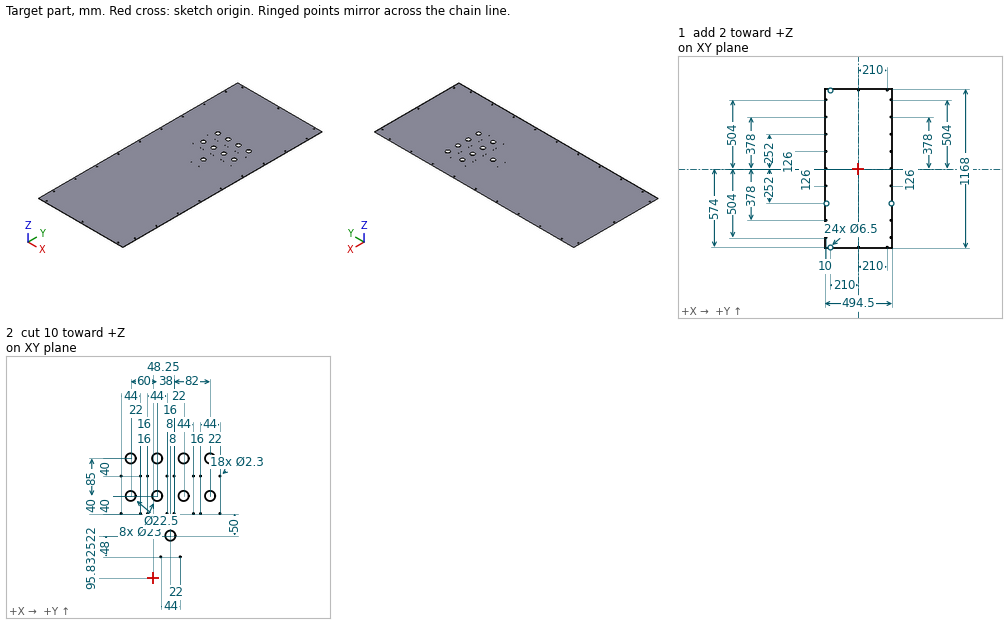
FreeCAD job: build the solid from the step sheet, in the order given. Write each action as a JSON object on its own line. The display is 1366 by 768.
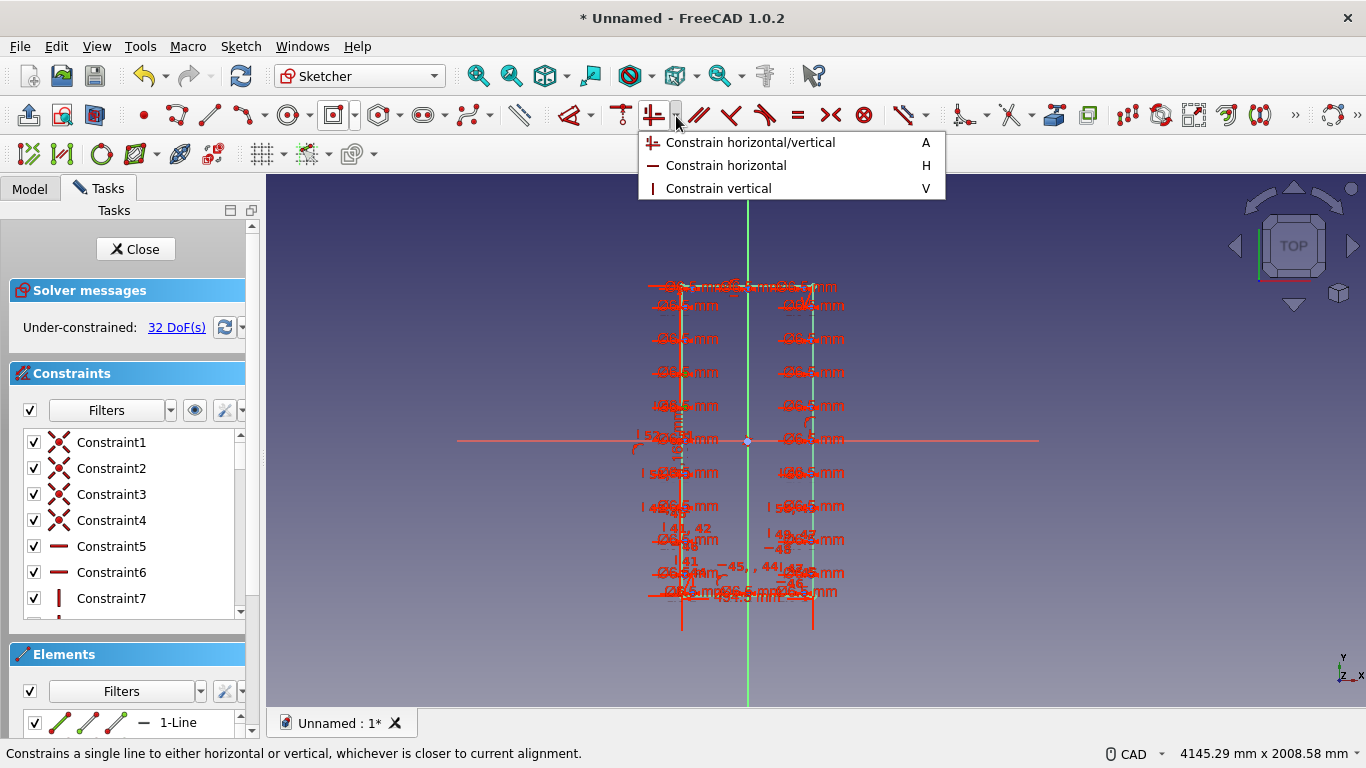
{"action": "left_click", "coordinate": [792, 188]}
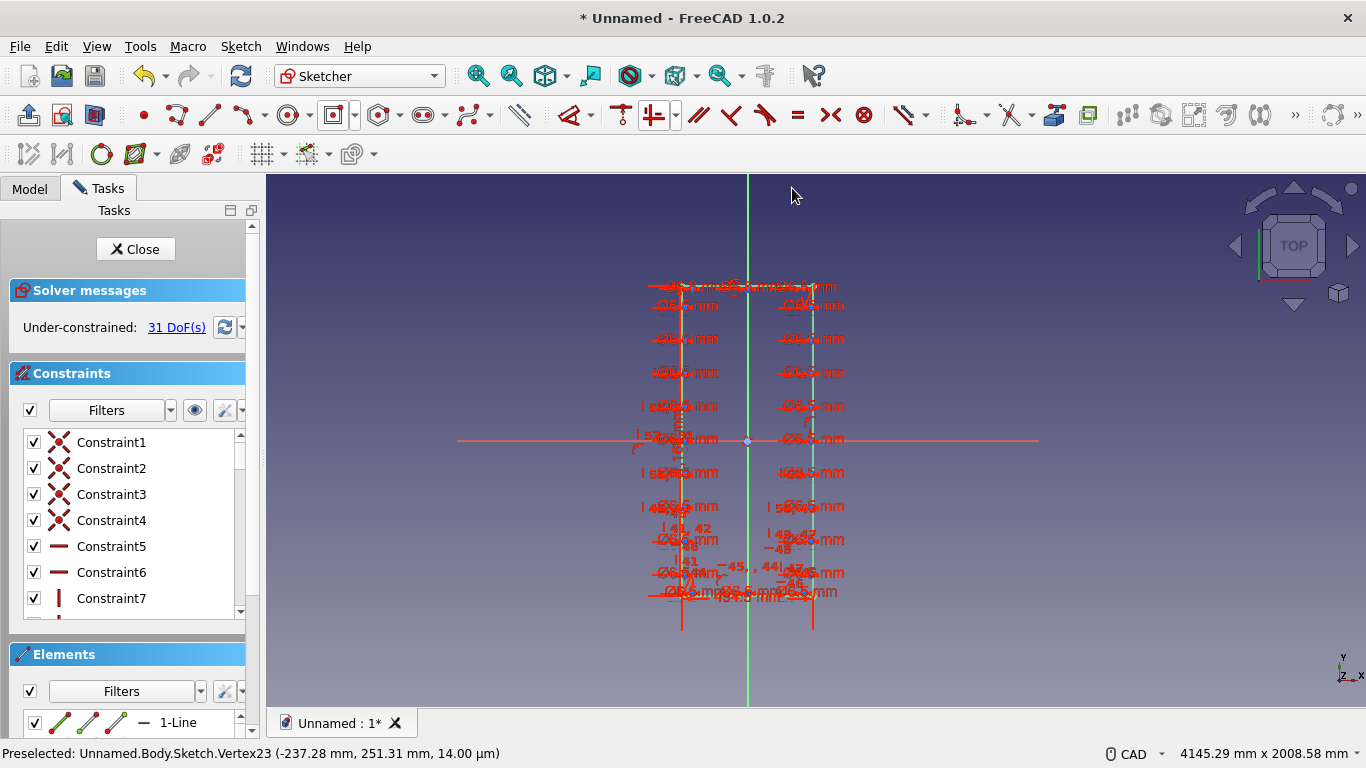
{"action": "left_click", "coordinate": [685, 374]}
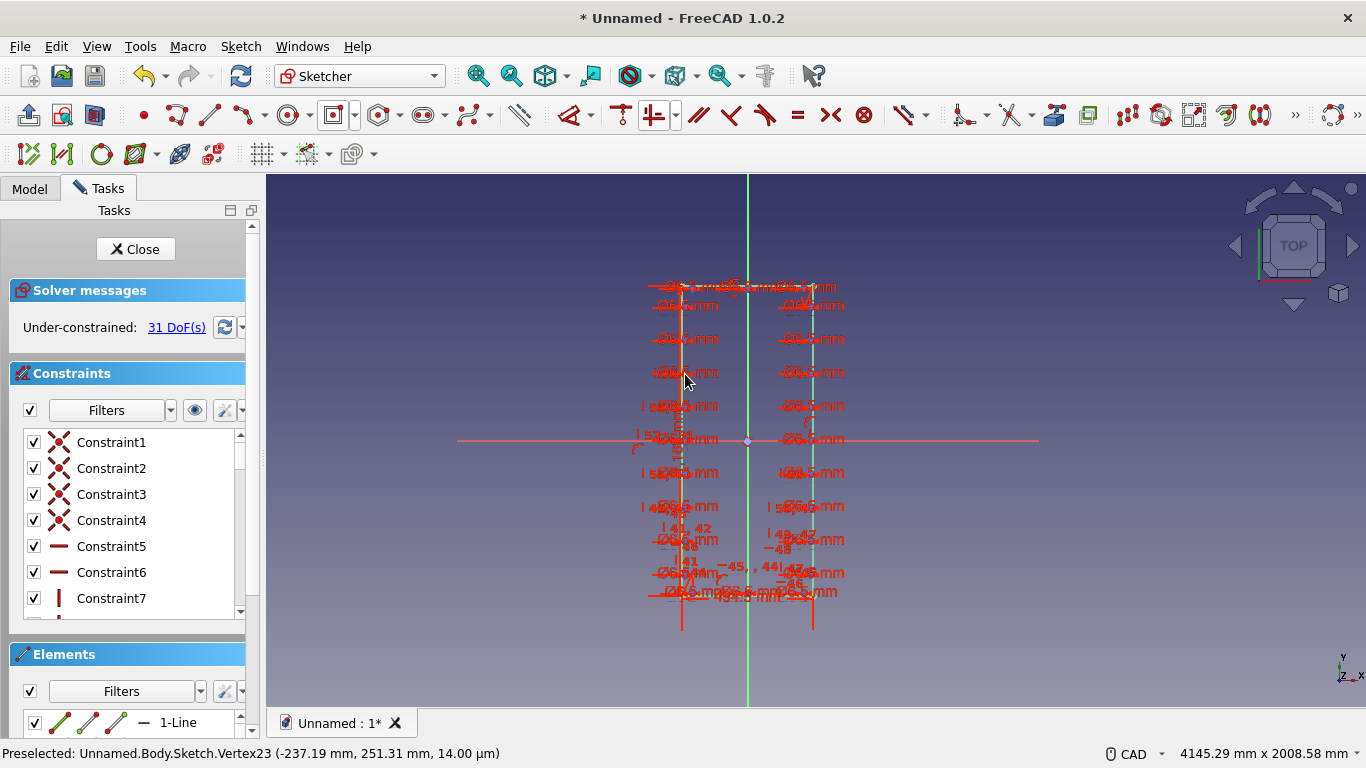
{"action": "left_click", "coordinate": [685, 341]}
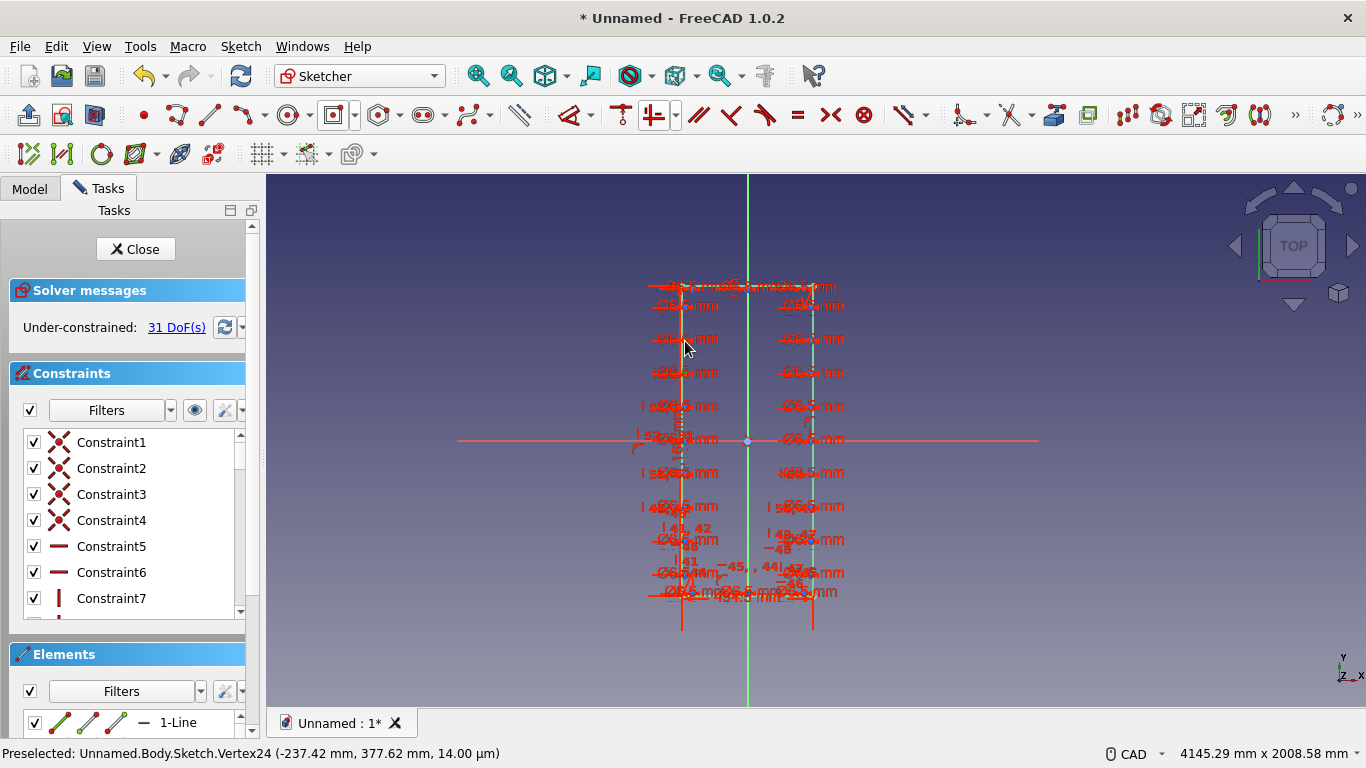
{"action": "key", "text": "v"}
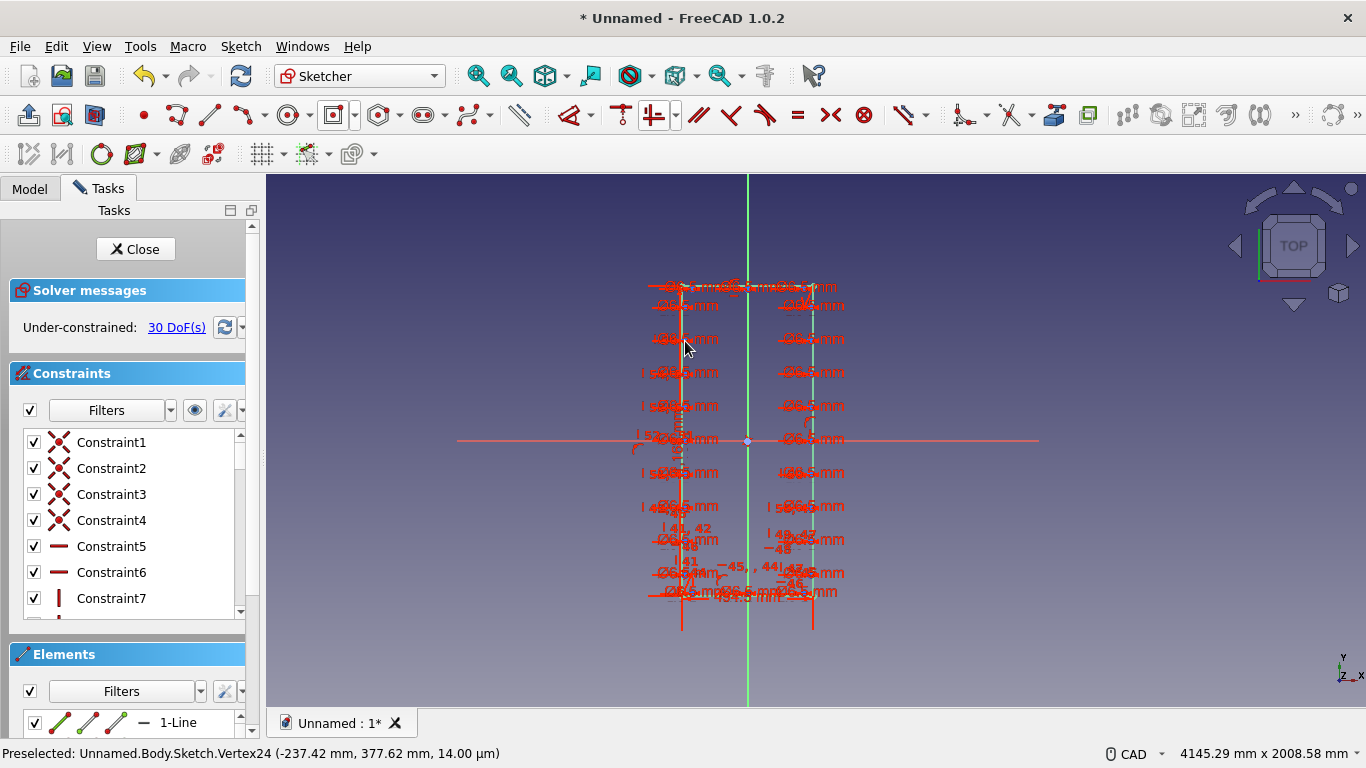
{"action": "left_click", "coordinate": [685, 341]}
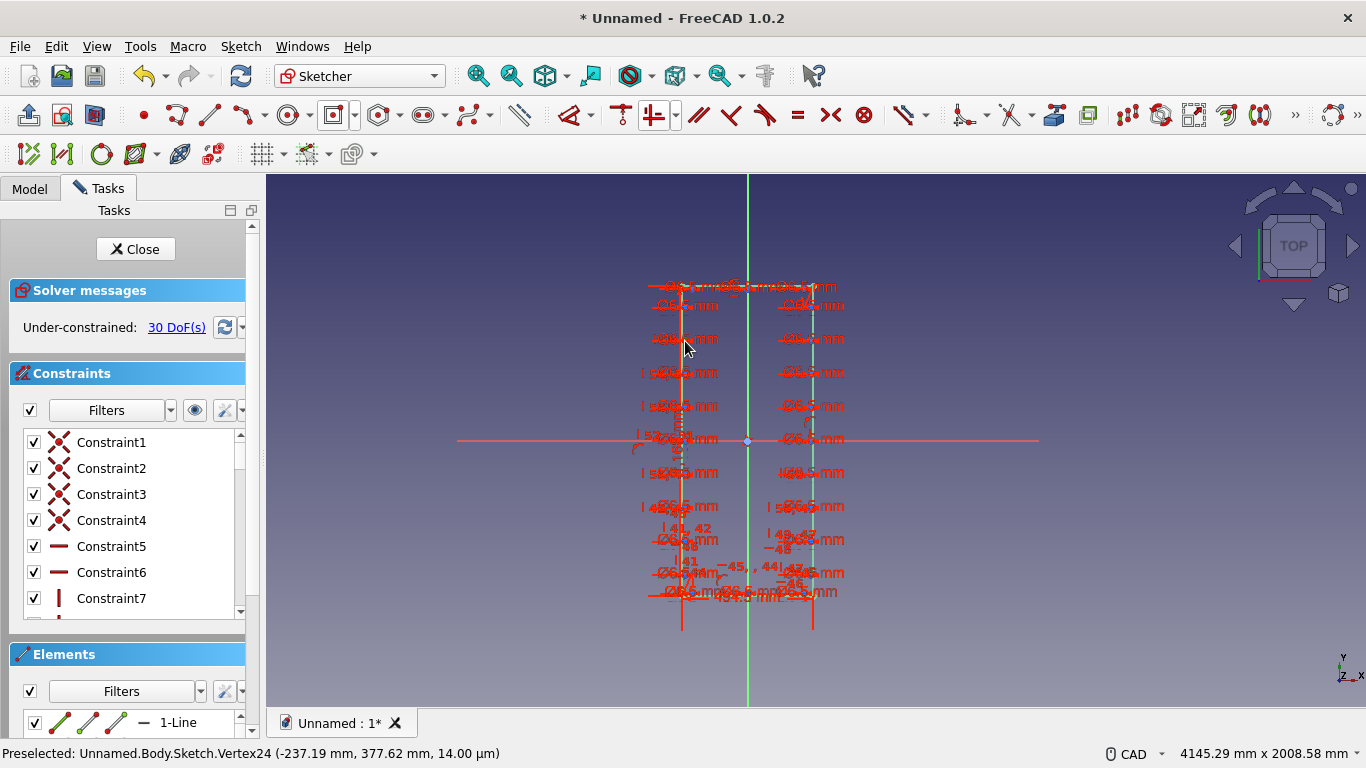
{"action": "left_click", "coordinate": [685, 308]}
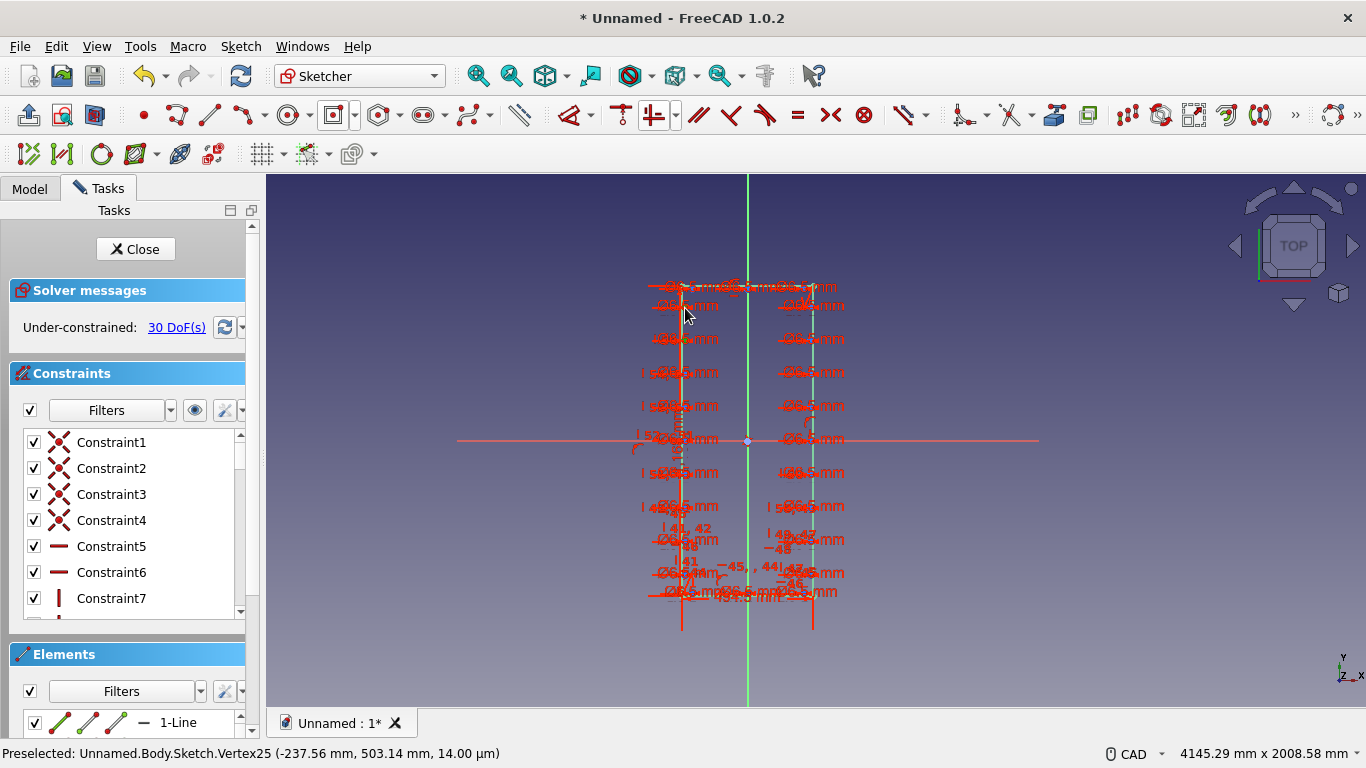
{"action": "left_click", "coordinate": [676, 116]}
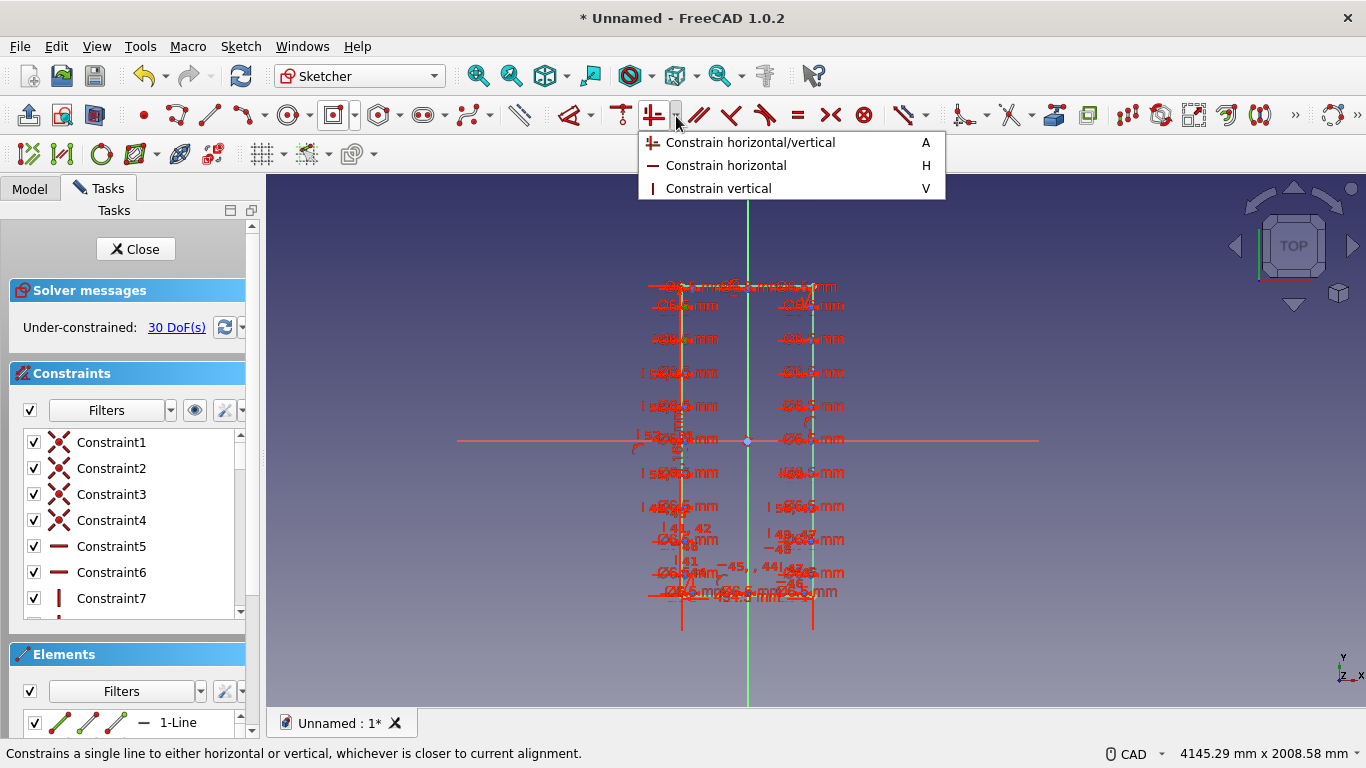
{"action": "left_click", "coordinate": [792, 188]}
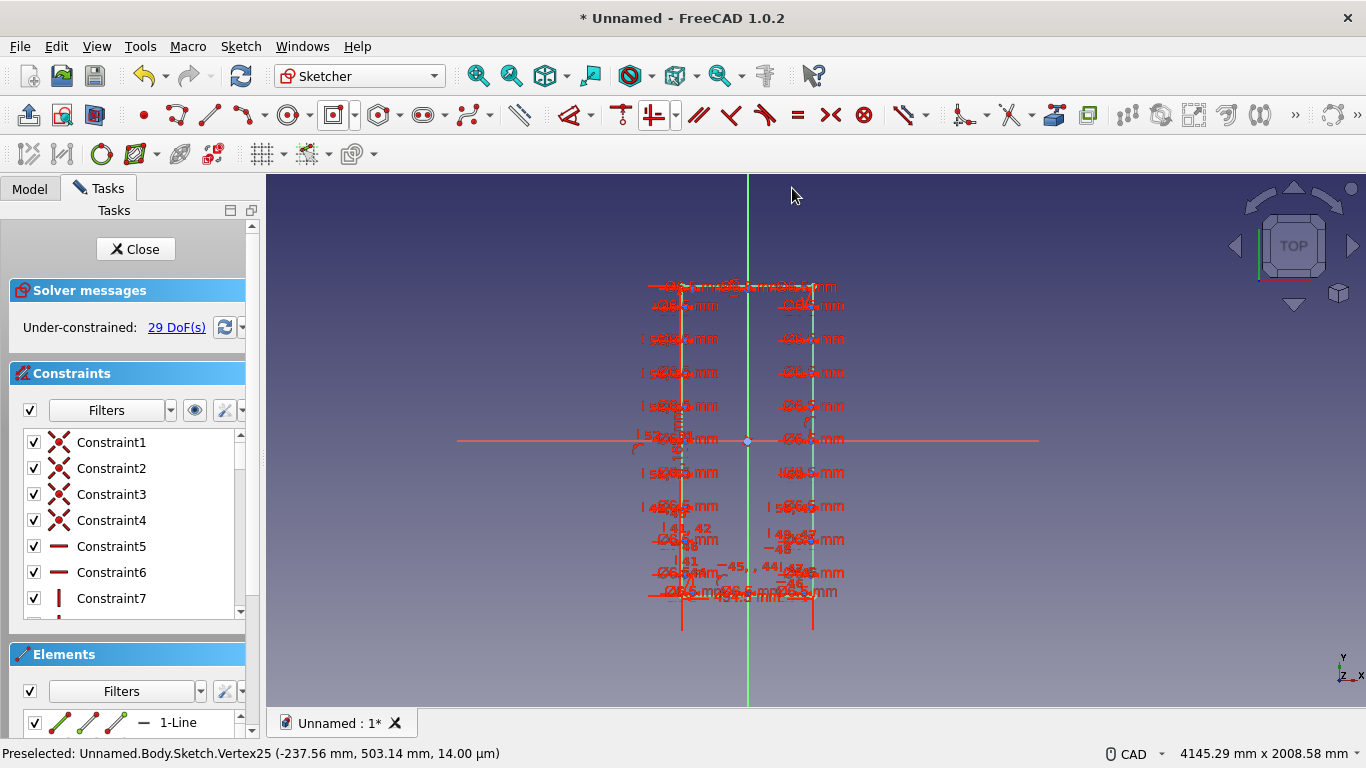
{"action": "left_click", "coordinate": [811, 475]}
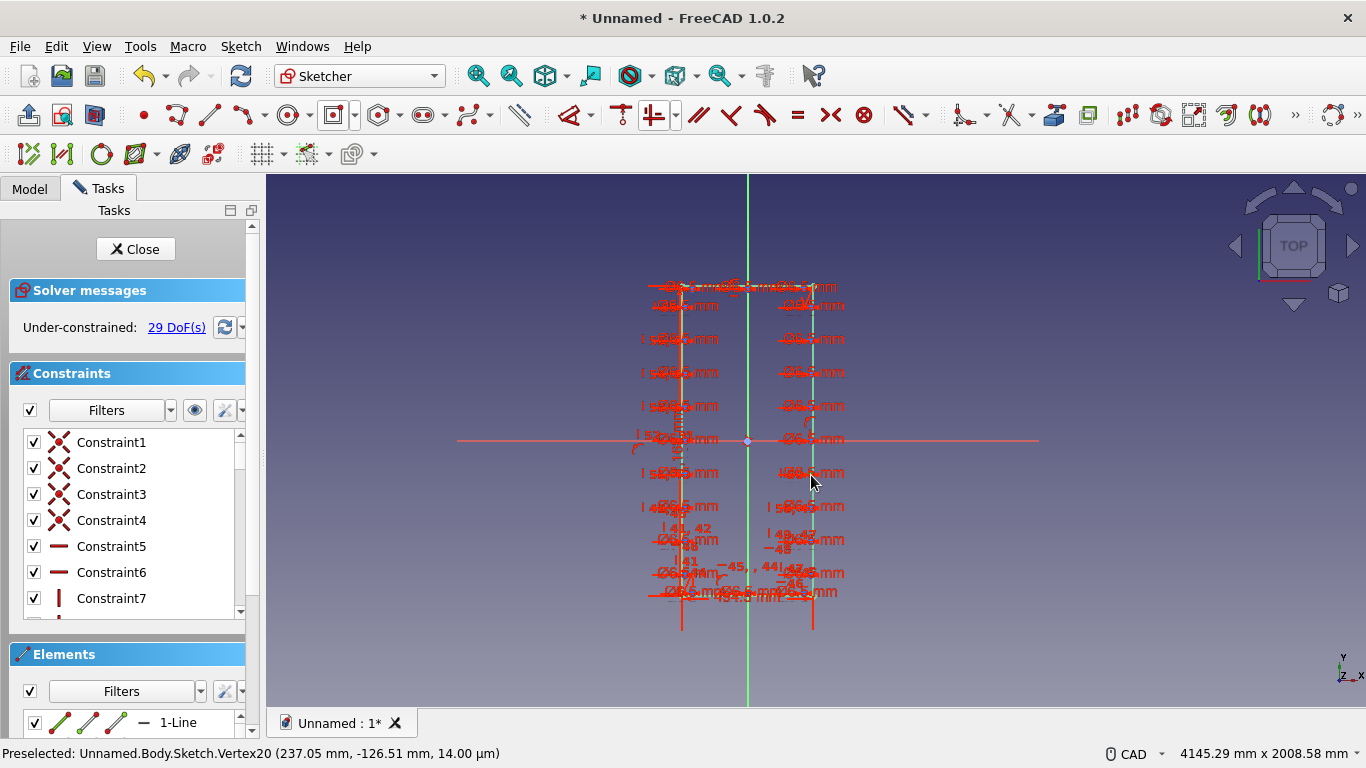
{"action": "left_click", "coordinate": [811, 441]}